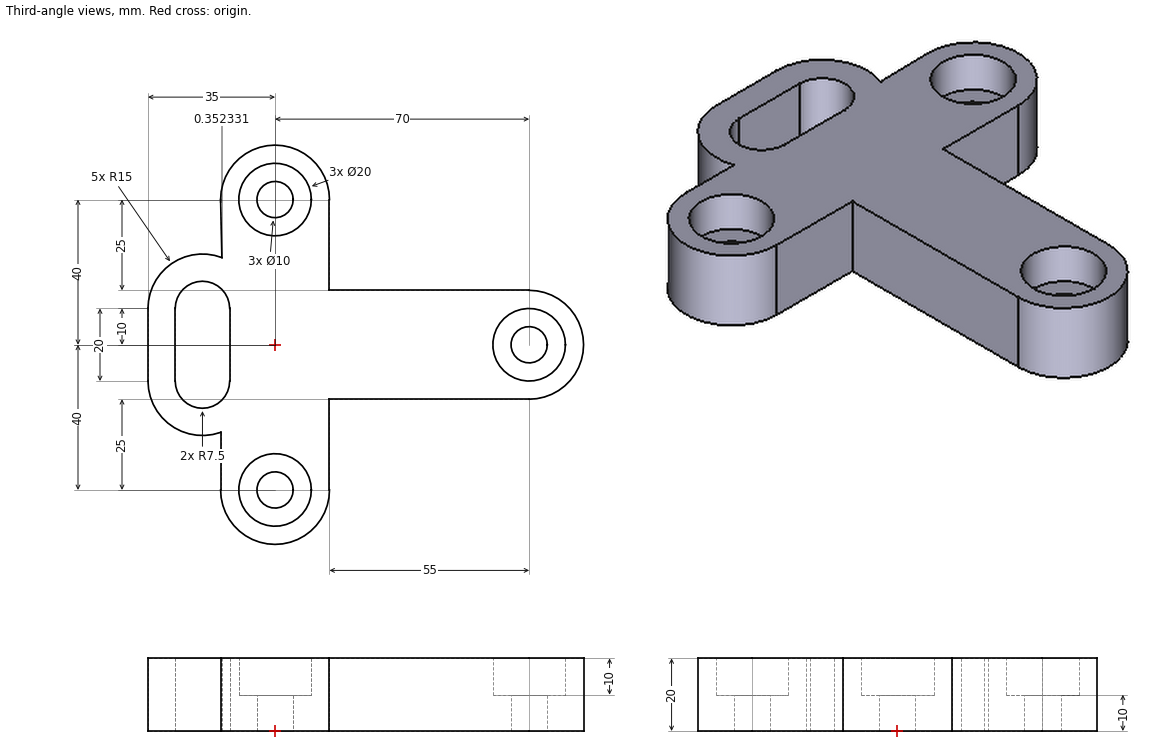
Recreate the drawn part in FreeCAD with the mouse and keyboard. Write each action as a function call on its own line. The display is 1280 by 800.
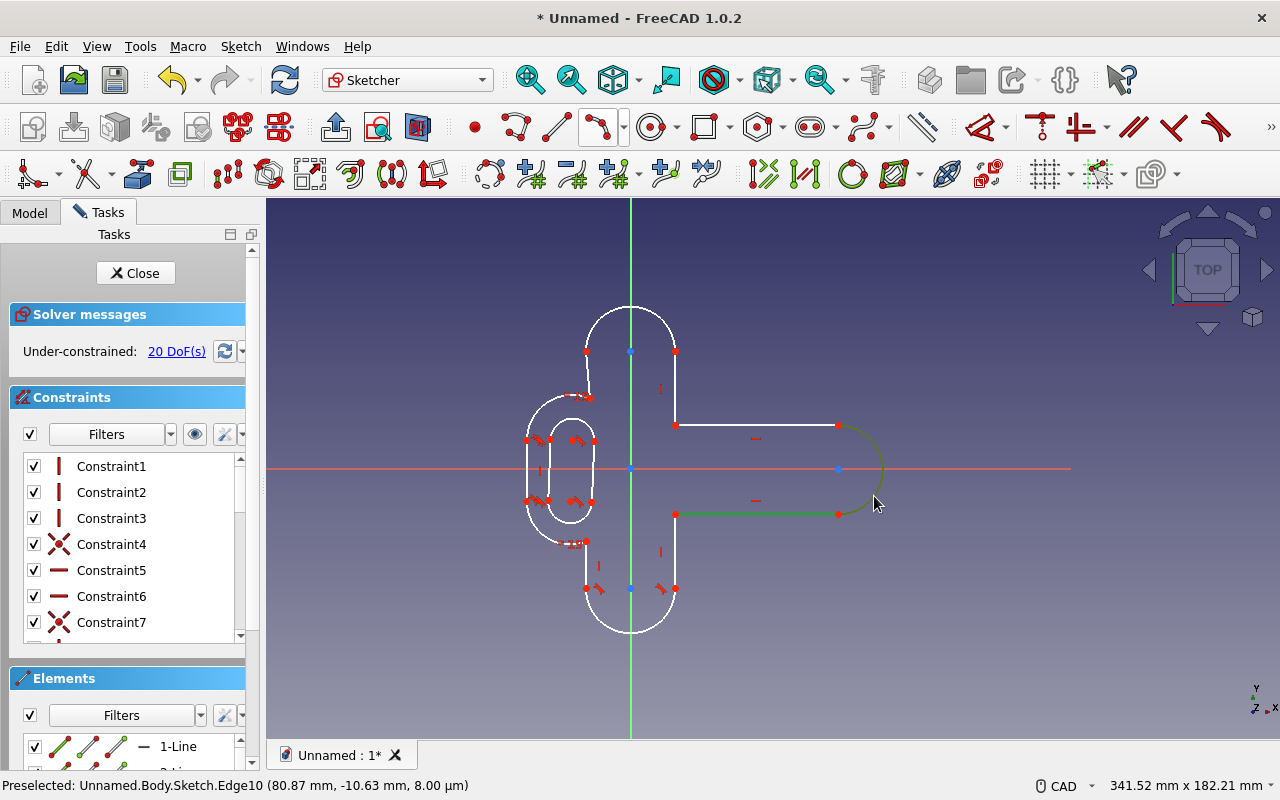
click(1216, 128)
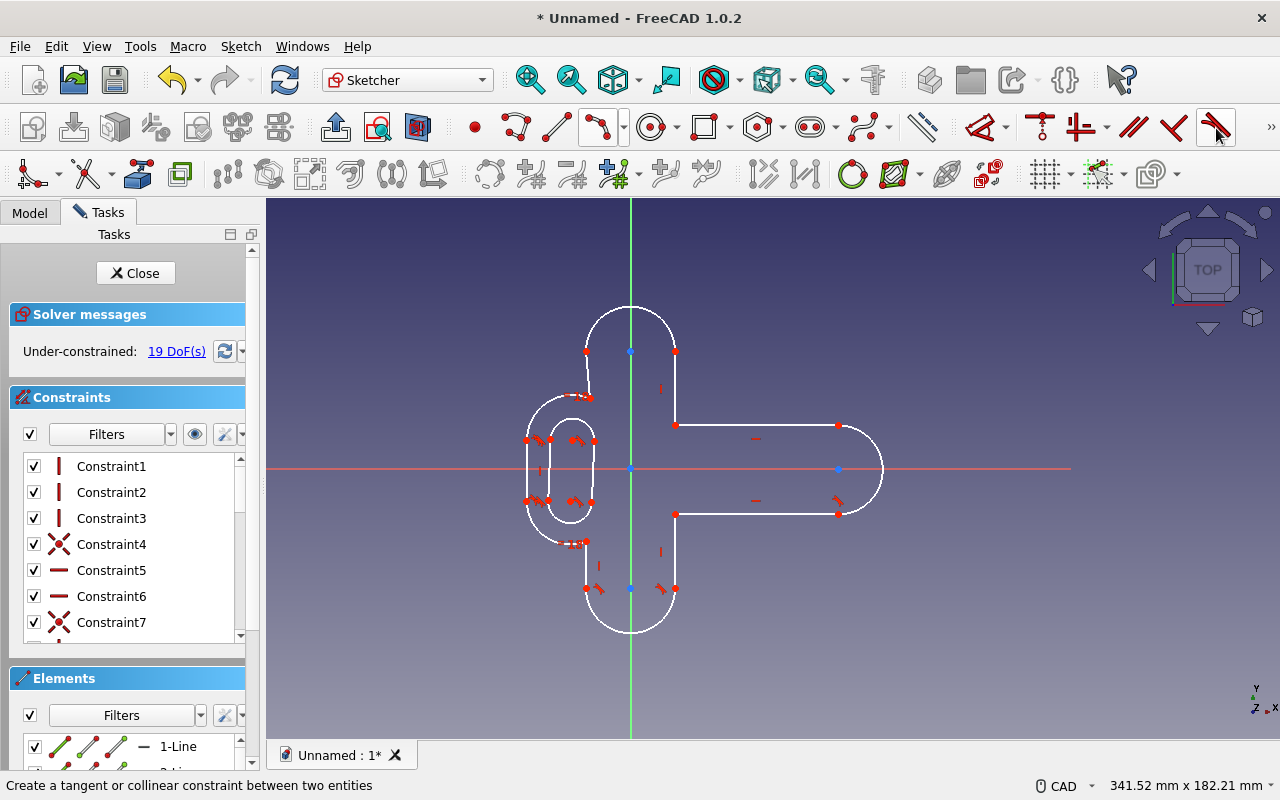
click(789, 425)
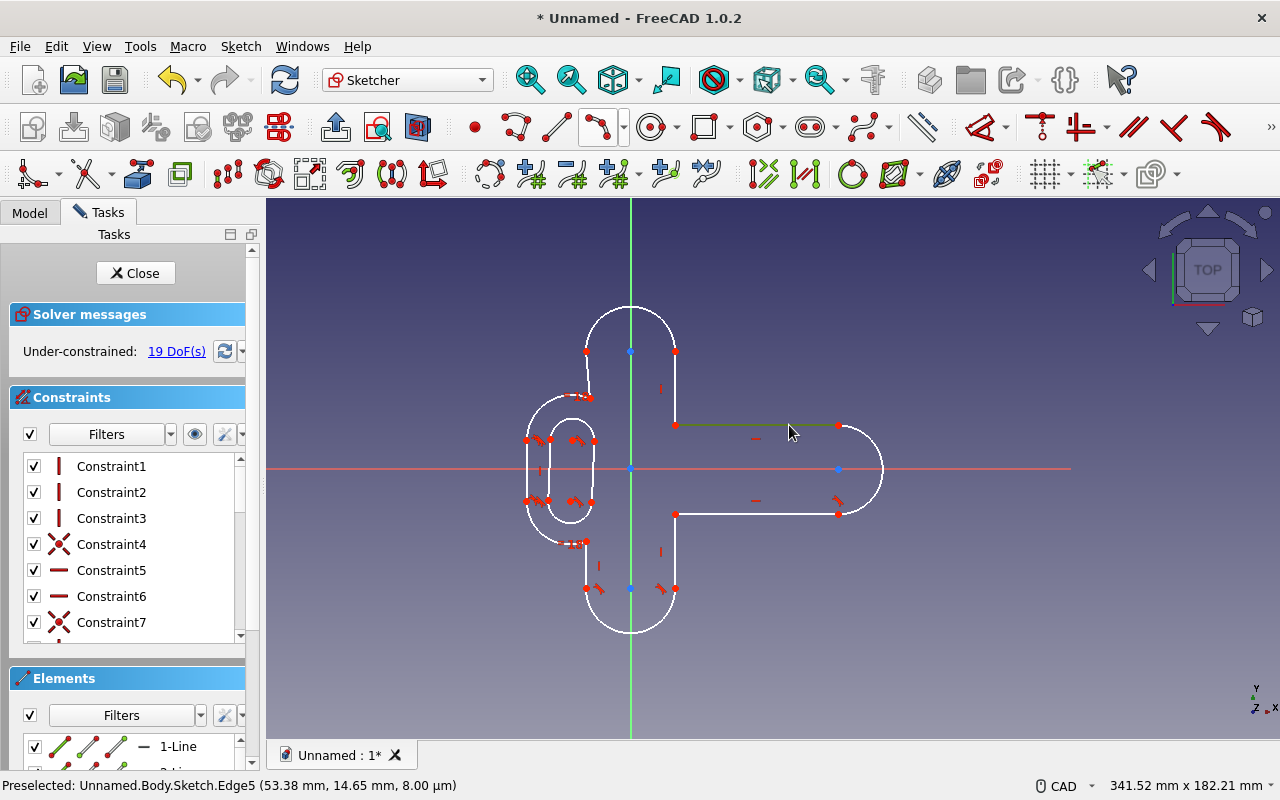
click(874, 496)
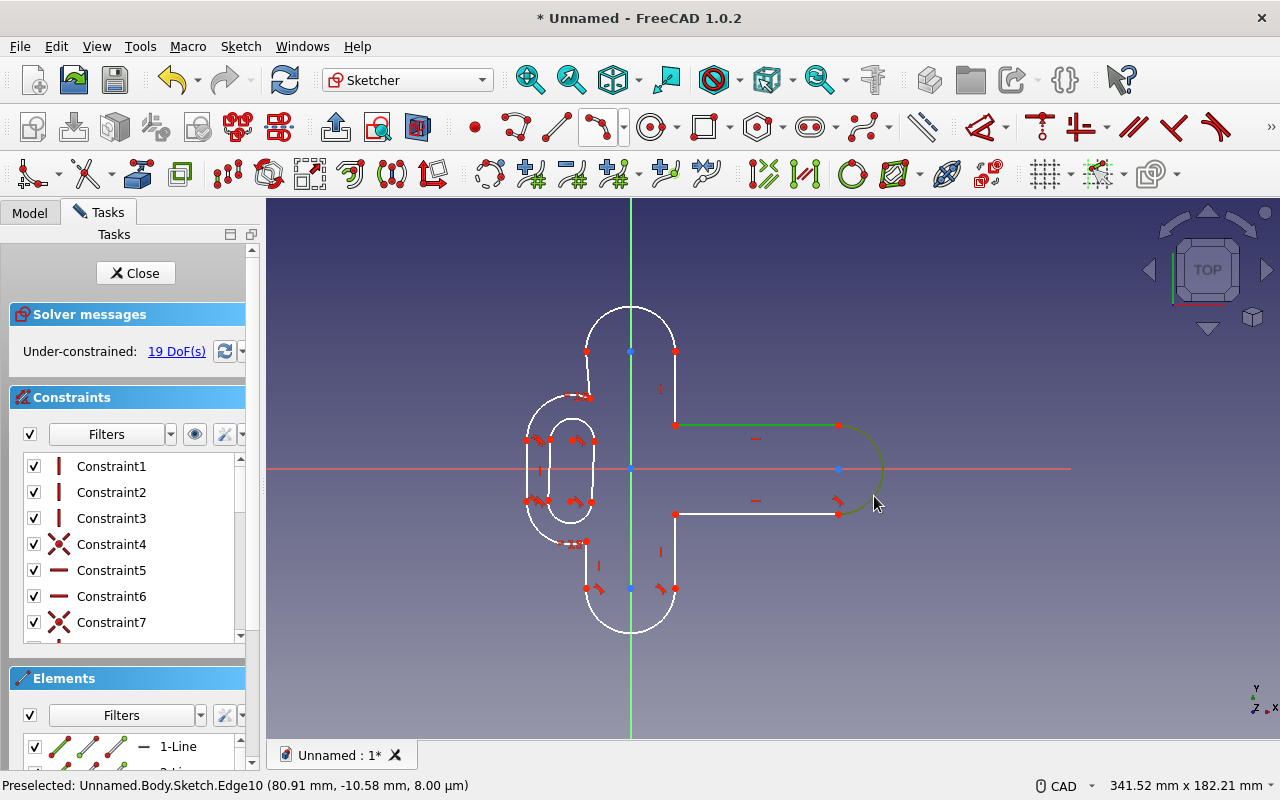
click(1216, 128)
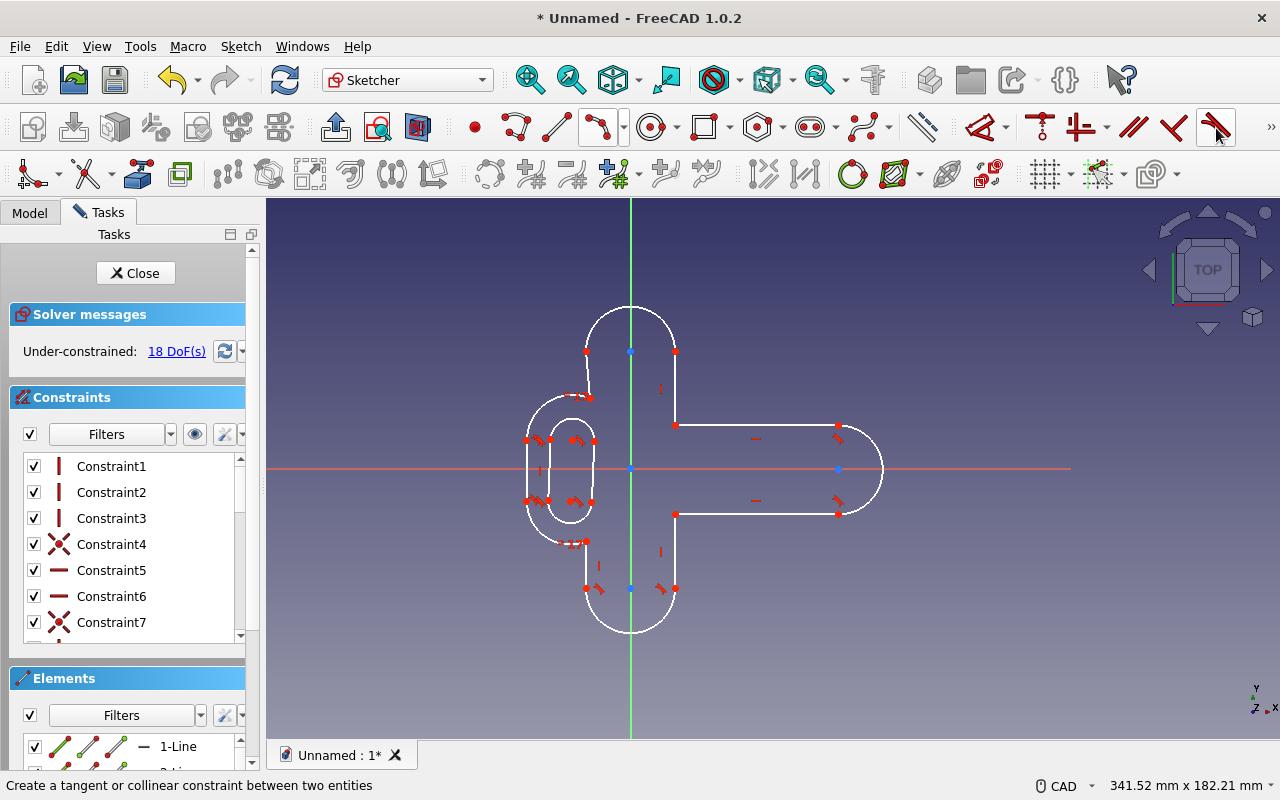
click(675, 403)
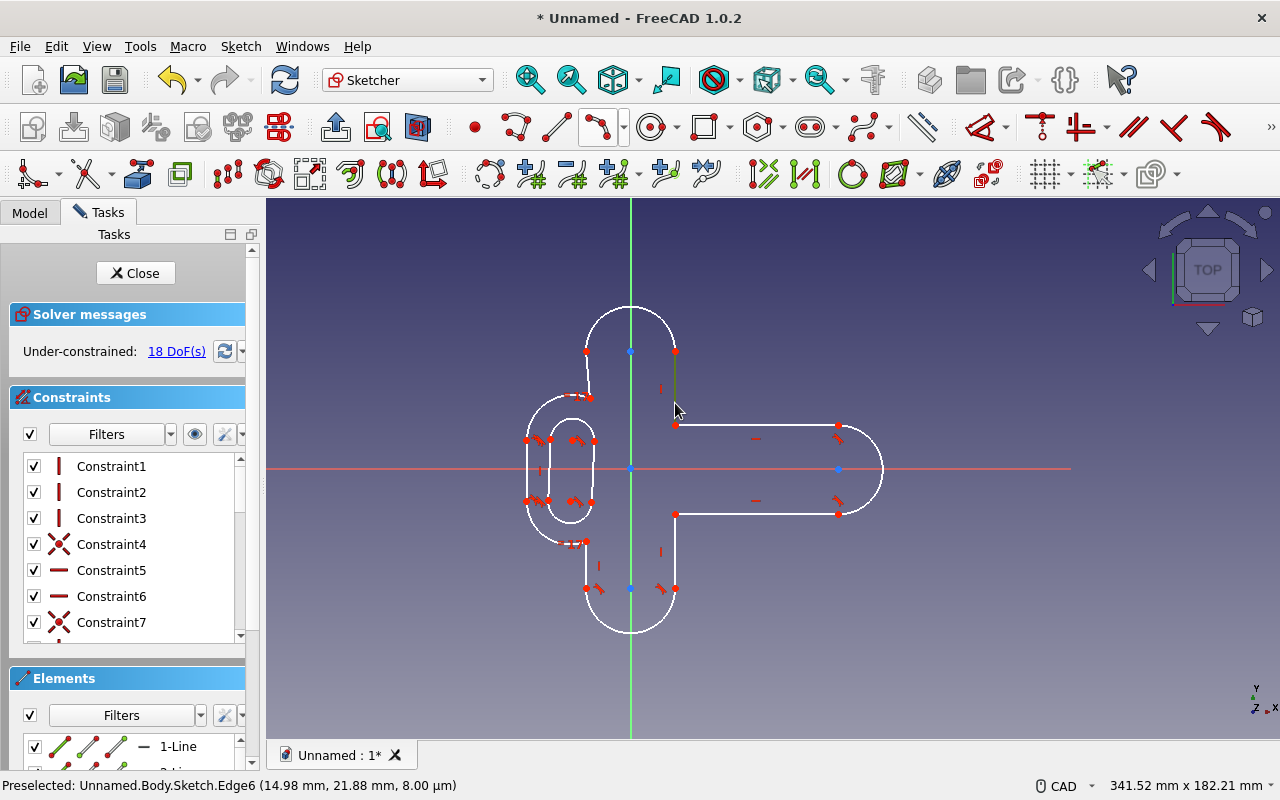
click(657, 315)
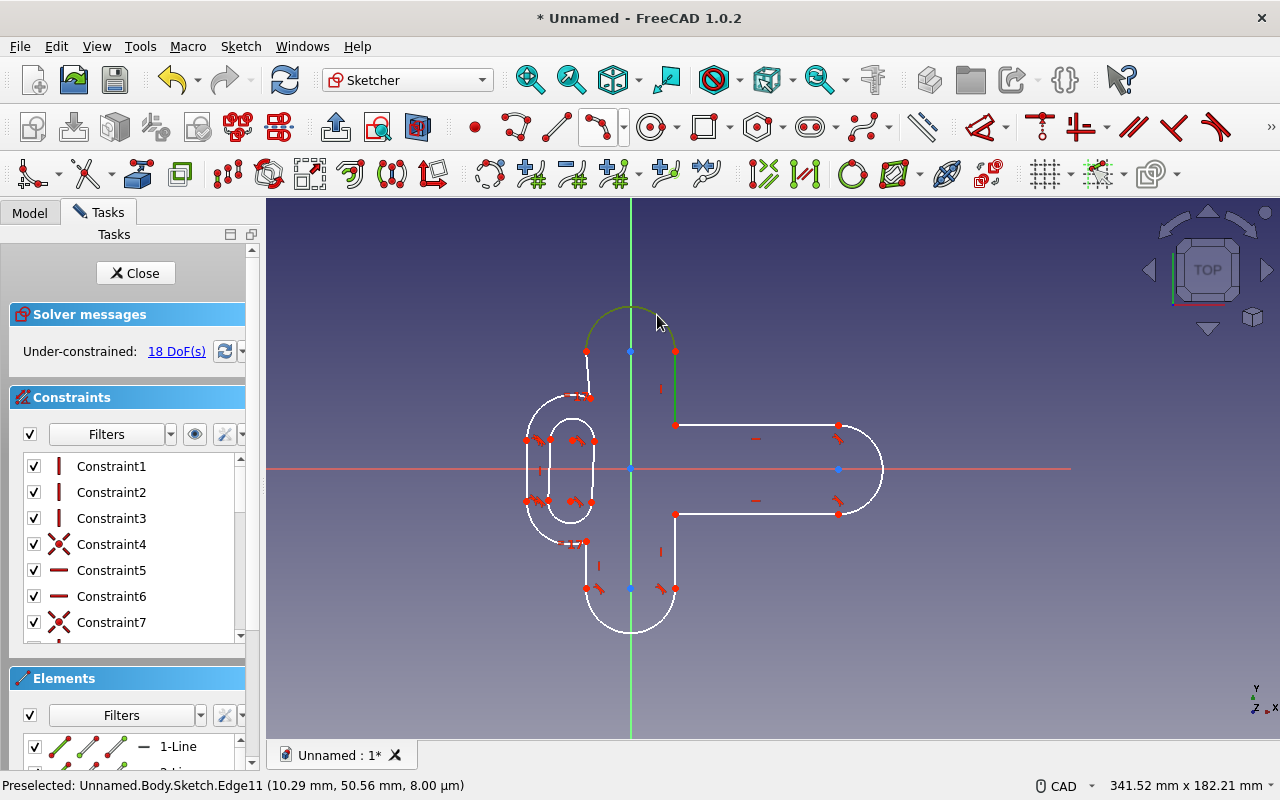
click(1216, 128)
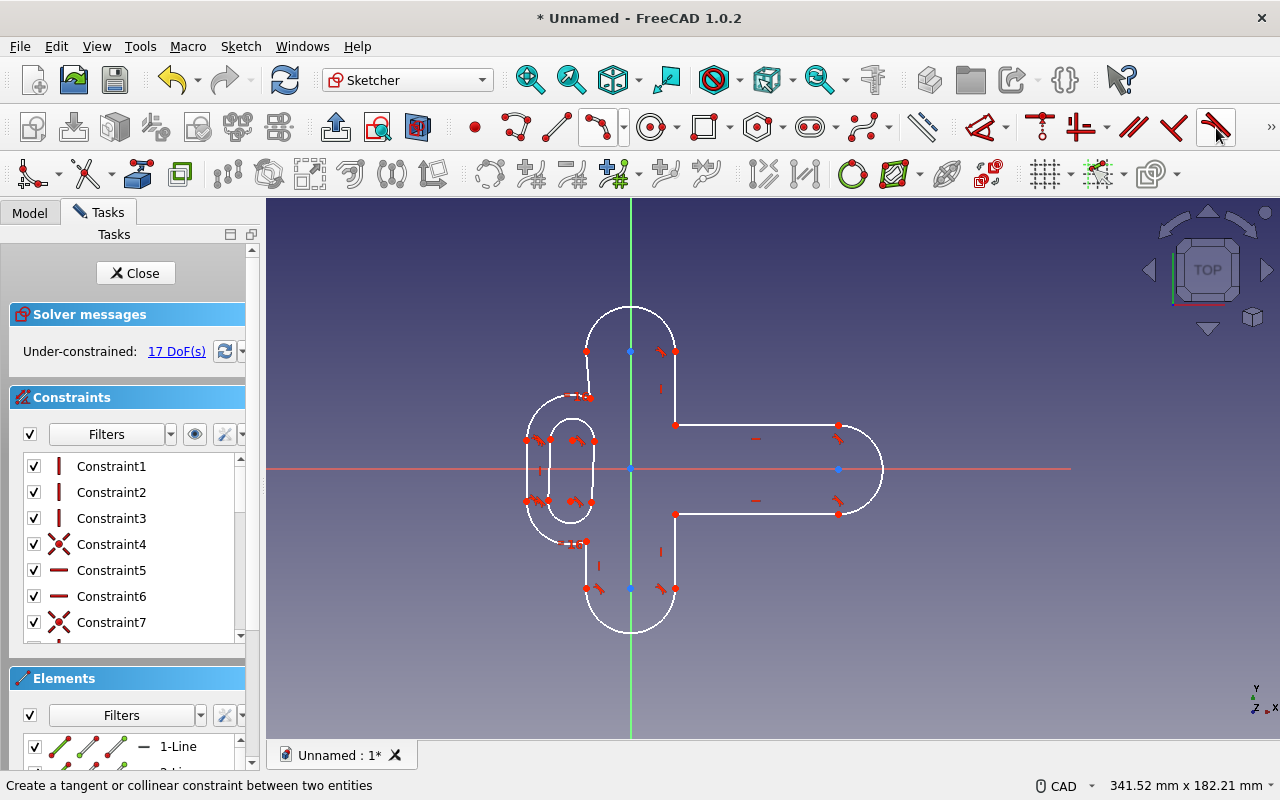
click(549, 482)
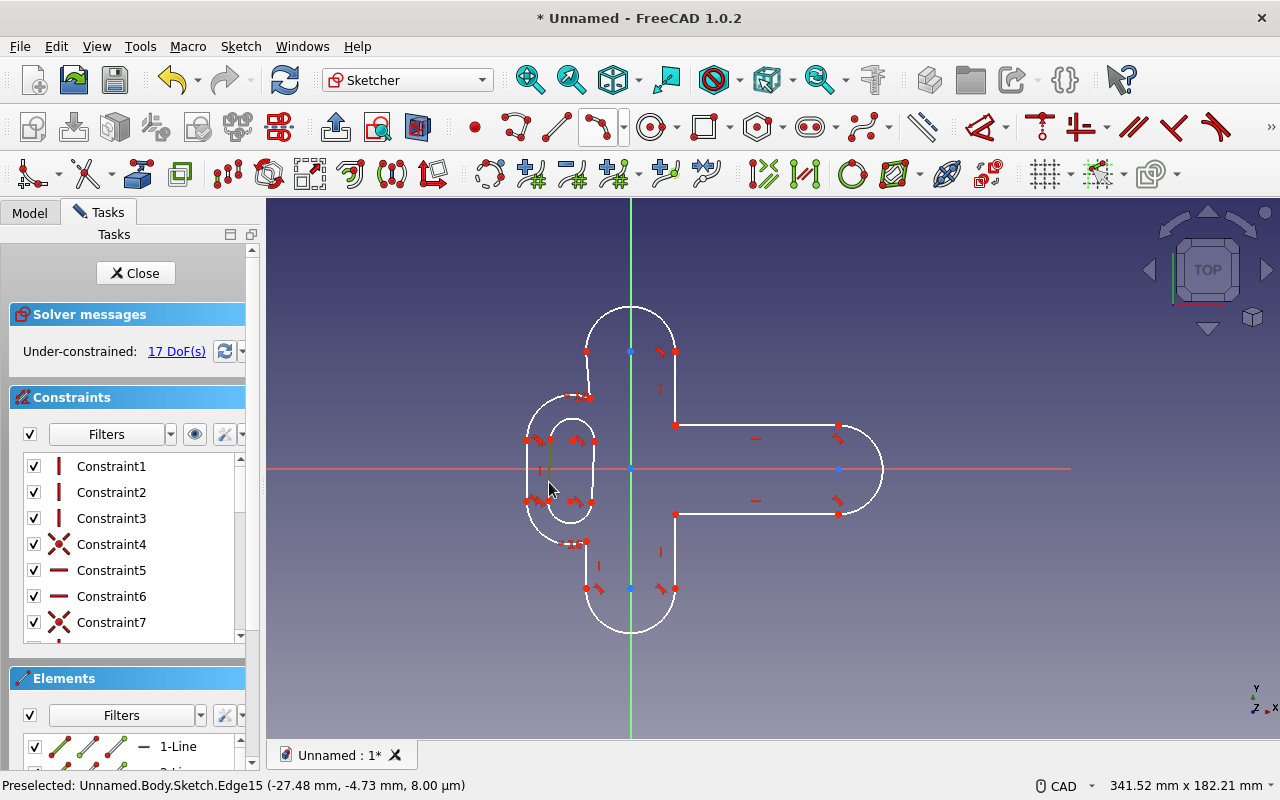
click(1106, 128)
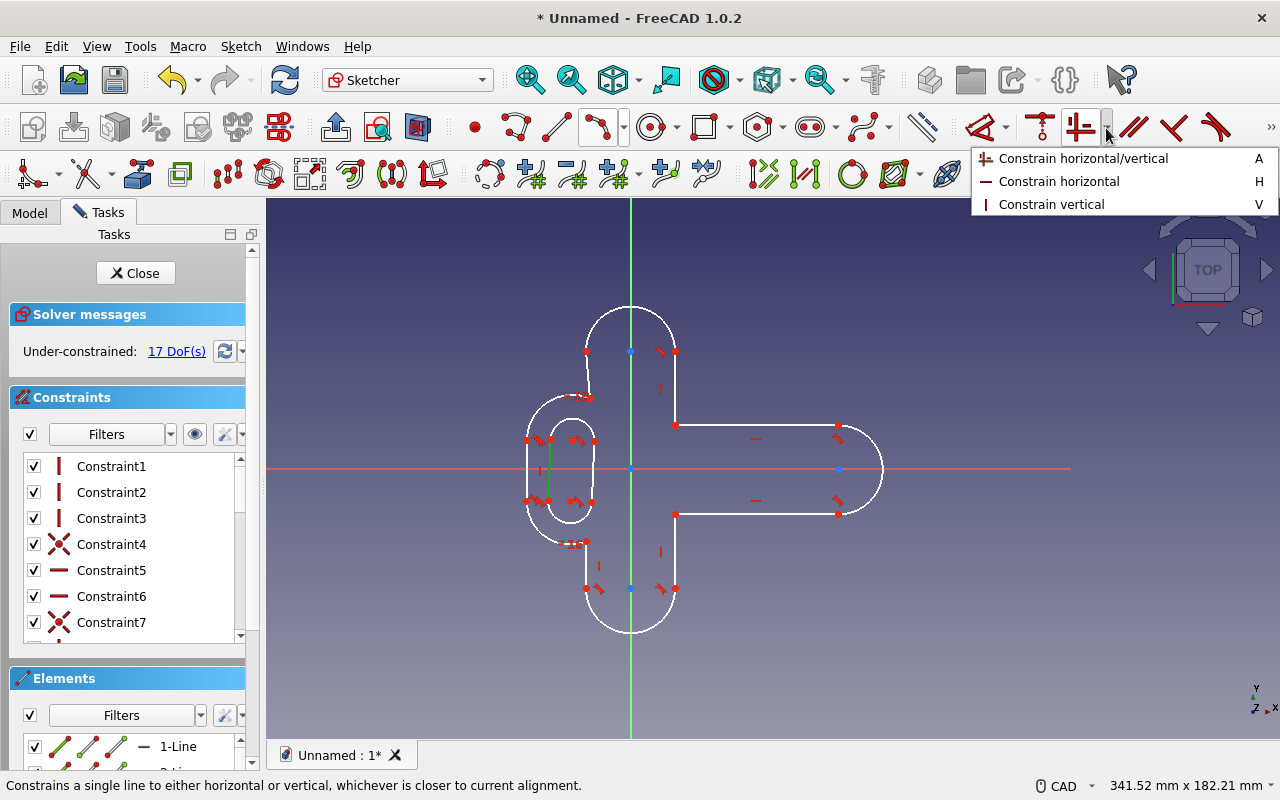
click(1125, 204)